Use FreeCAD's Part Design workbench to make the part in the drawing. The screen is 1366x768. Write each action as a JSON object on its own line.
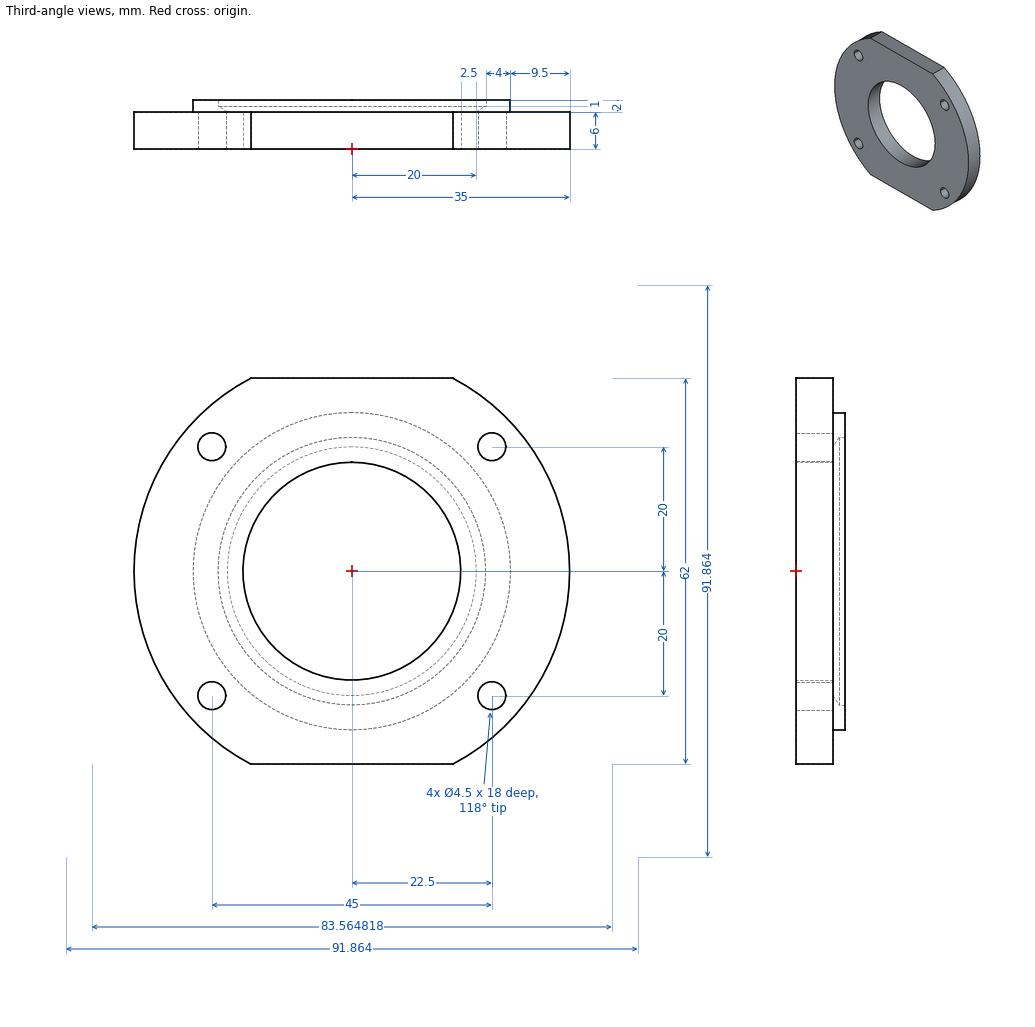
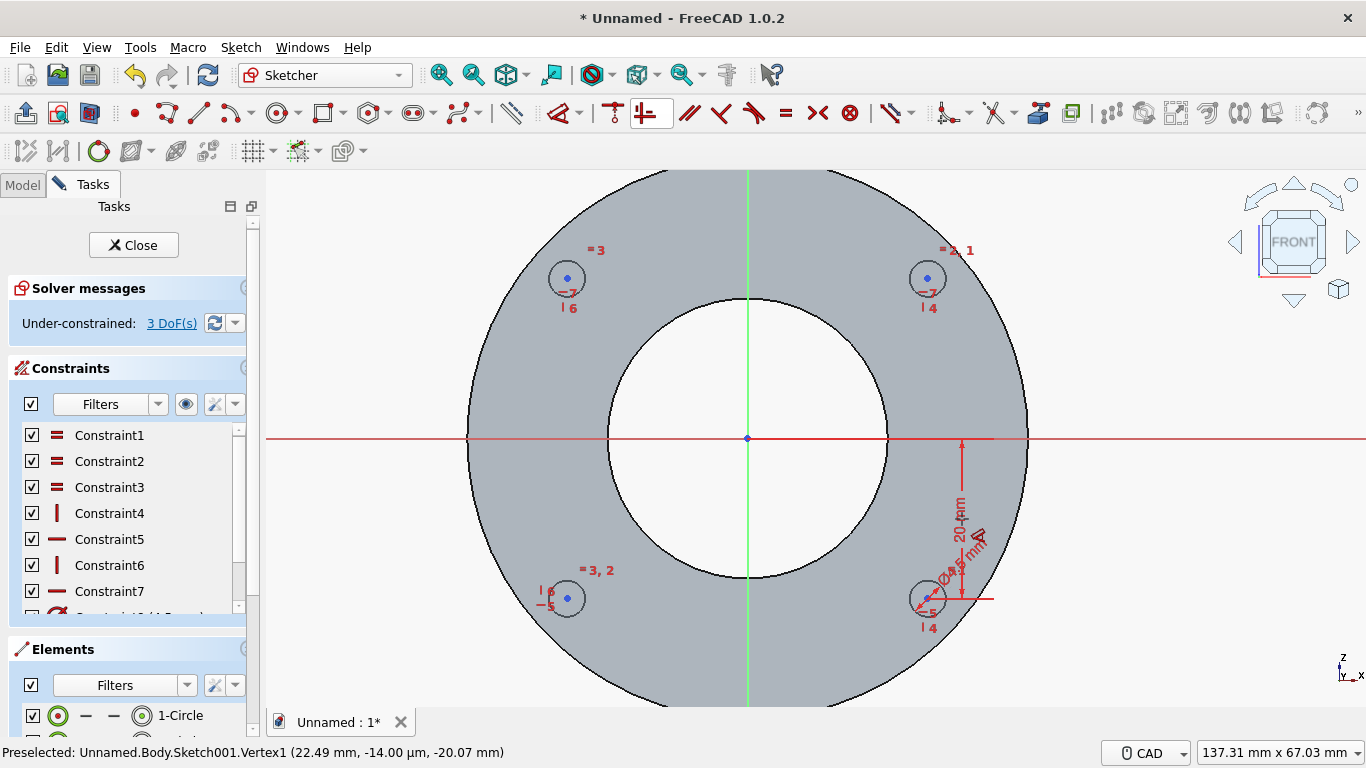
{"action": "left_click", "coordinate": [928, 279]}
{"action": "left_click", "coordinate": [962, 359]}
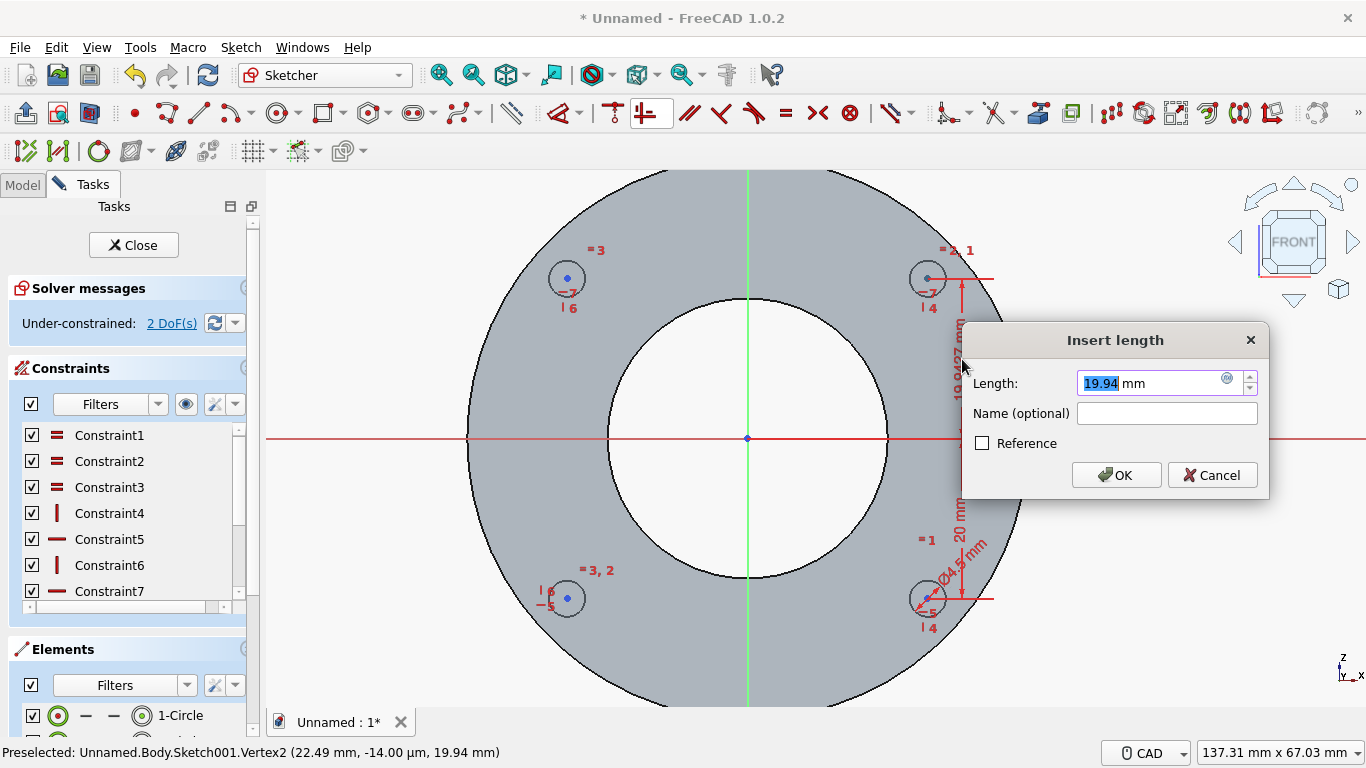
{"action": "type", "text": "20"}
{"action": "key", "text": "Return"}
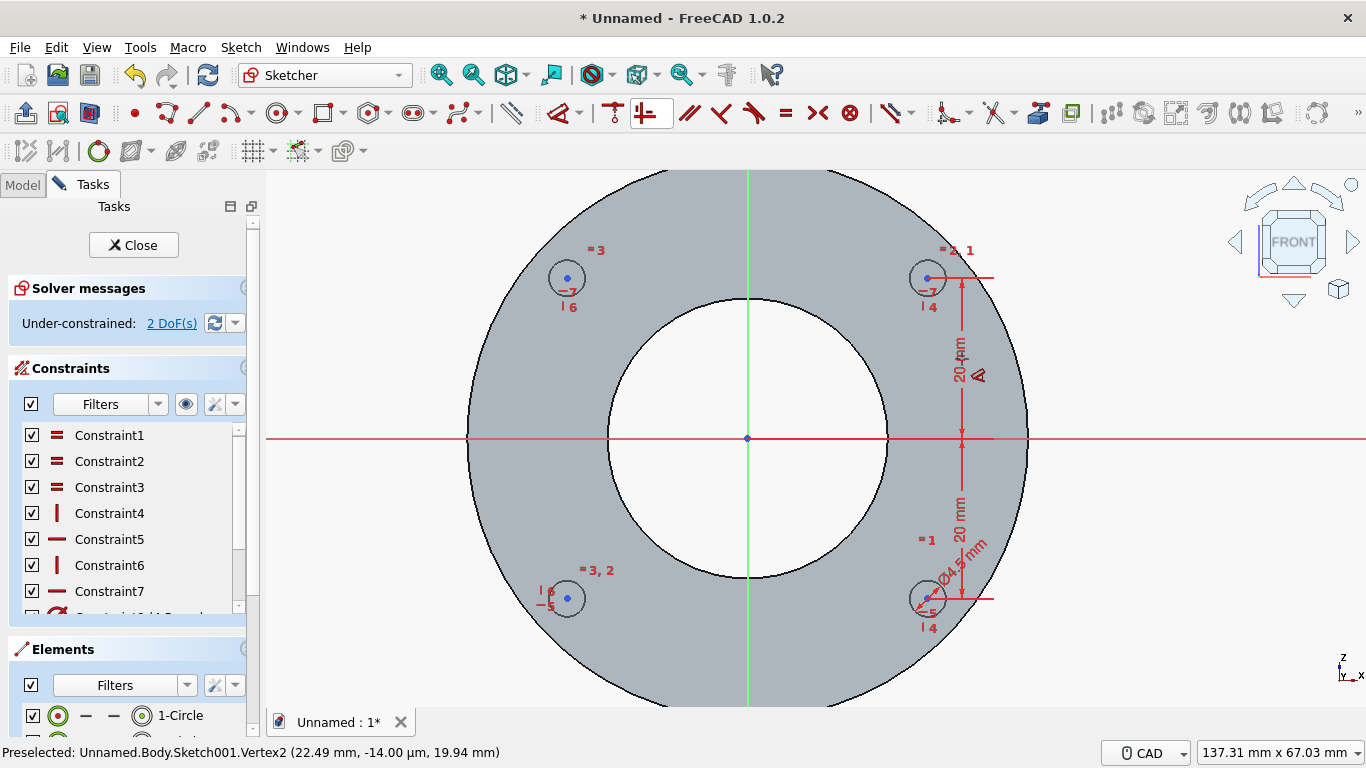
{"action": "left_click", "coordinate": [928, 599]}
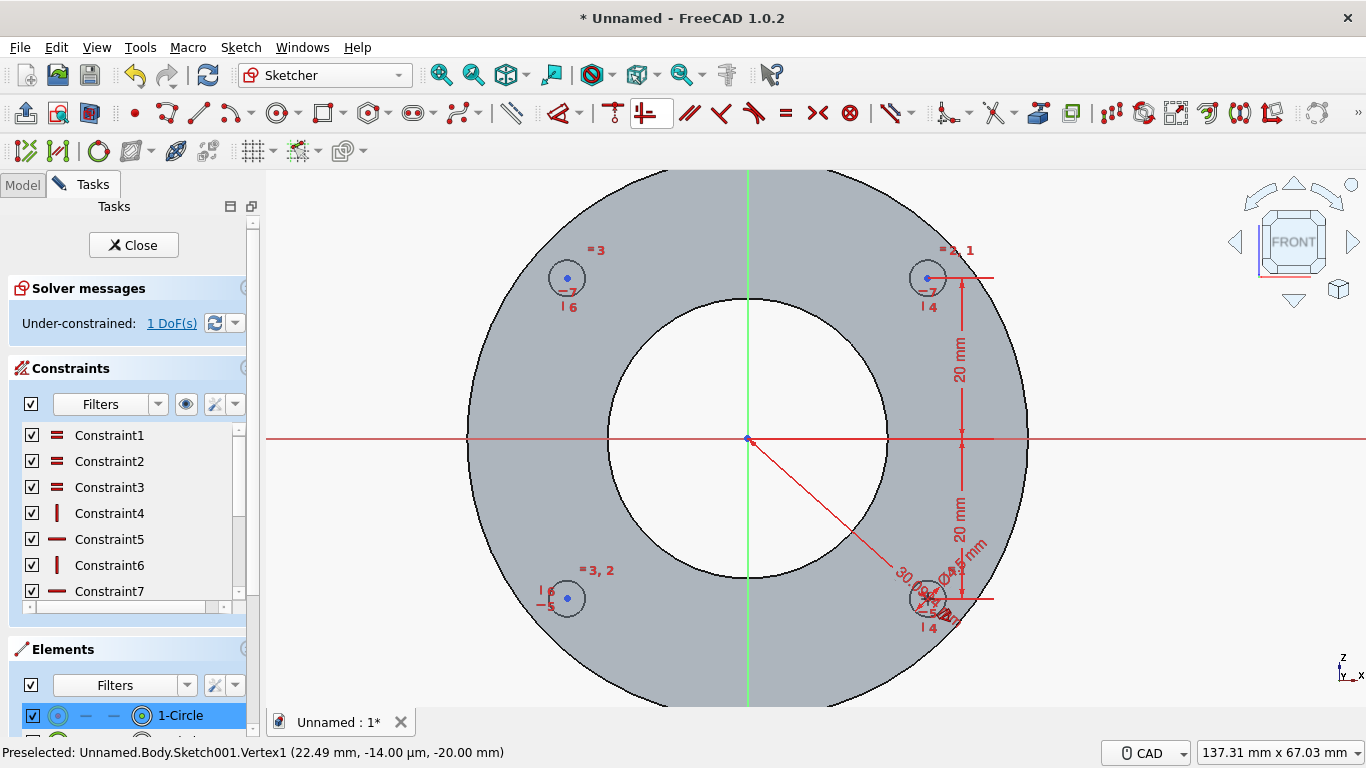
{"action": "left_click", "coordinate": [567, 599]}
{"action": "left_click", "coordinate": [664, 633]}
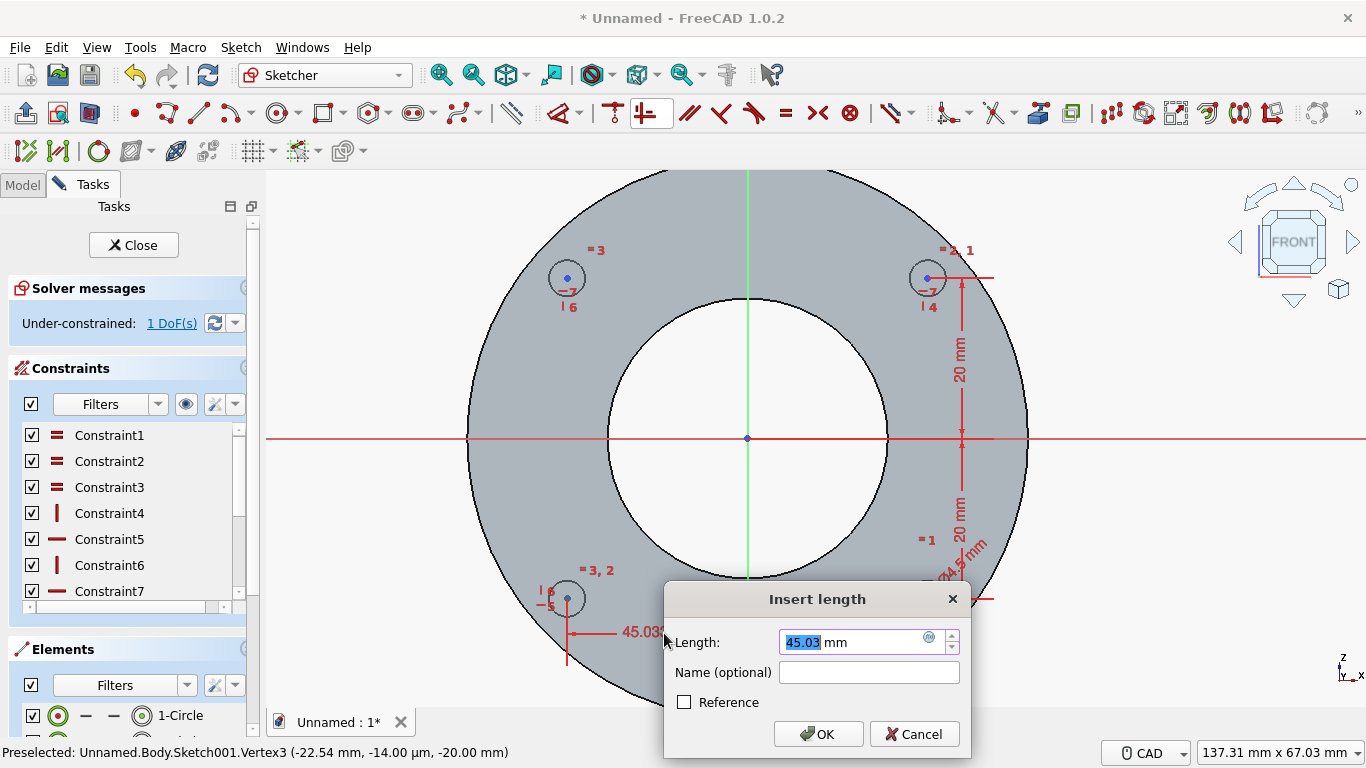
{"action": "type", "text": "45"}
{"action": "key", "text": "Return"}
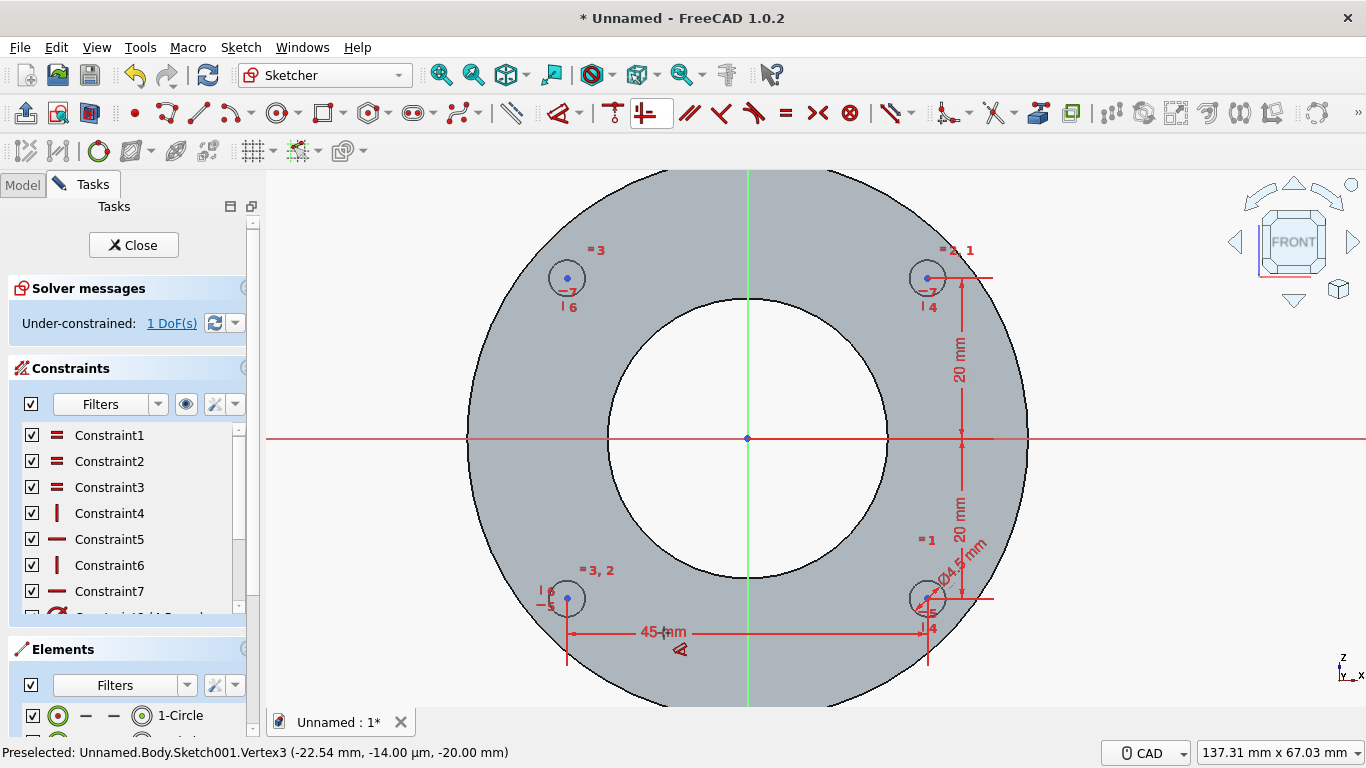
{"action": "left_click", "coordinate": [928, 599]}
{"action": "left_click", "coordinate": [838, 633]}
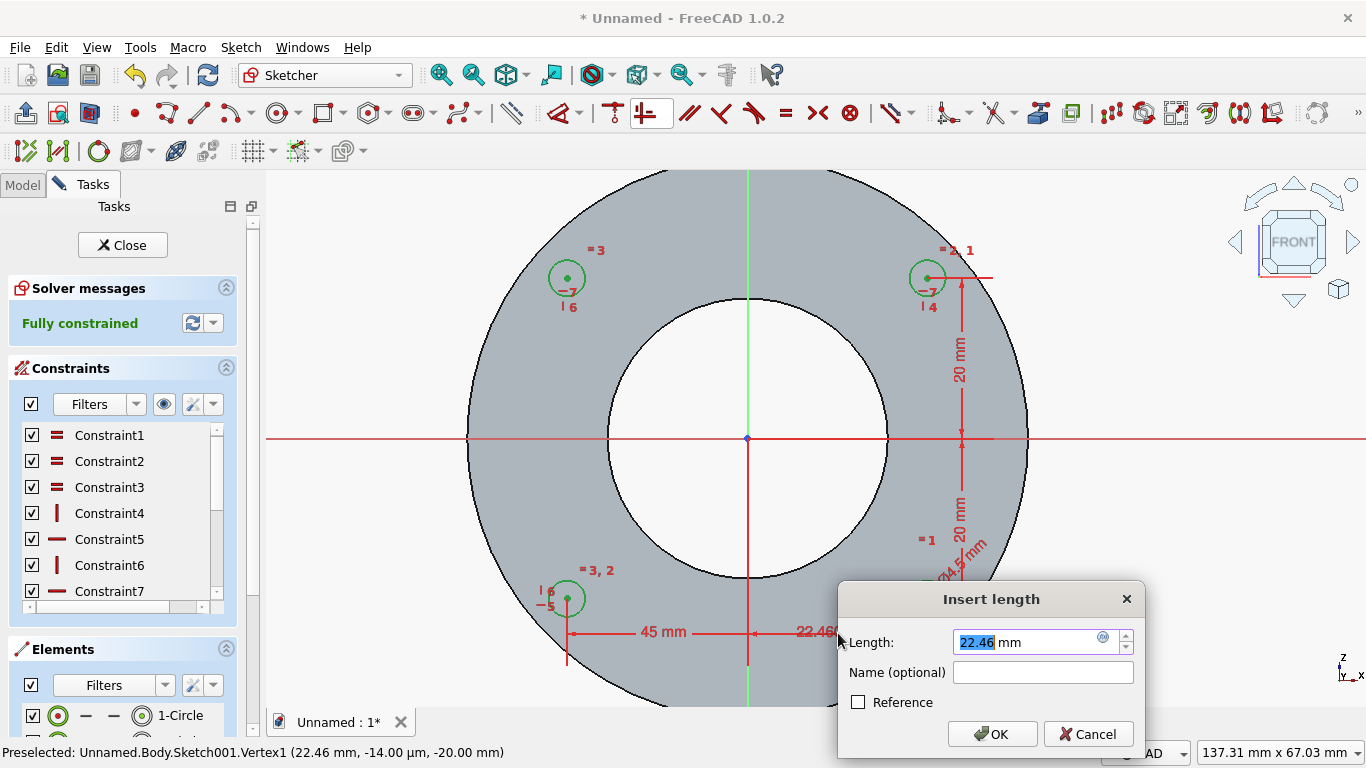
{"action": "type", "text": "22.5"}
{"action": "key", "text": "Return"}
{"action": "key", "text": "Escape"}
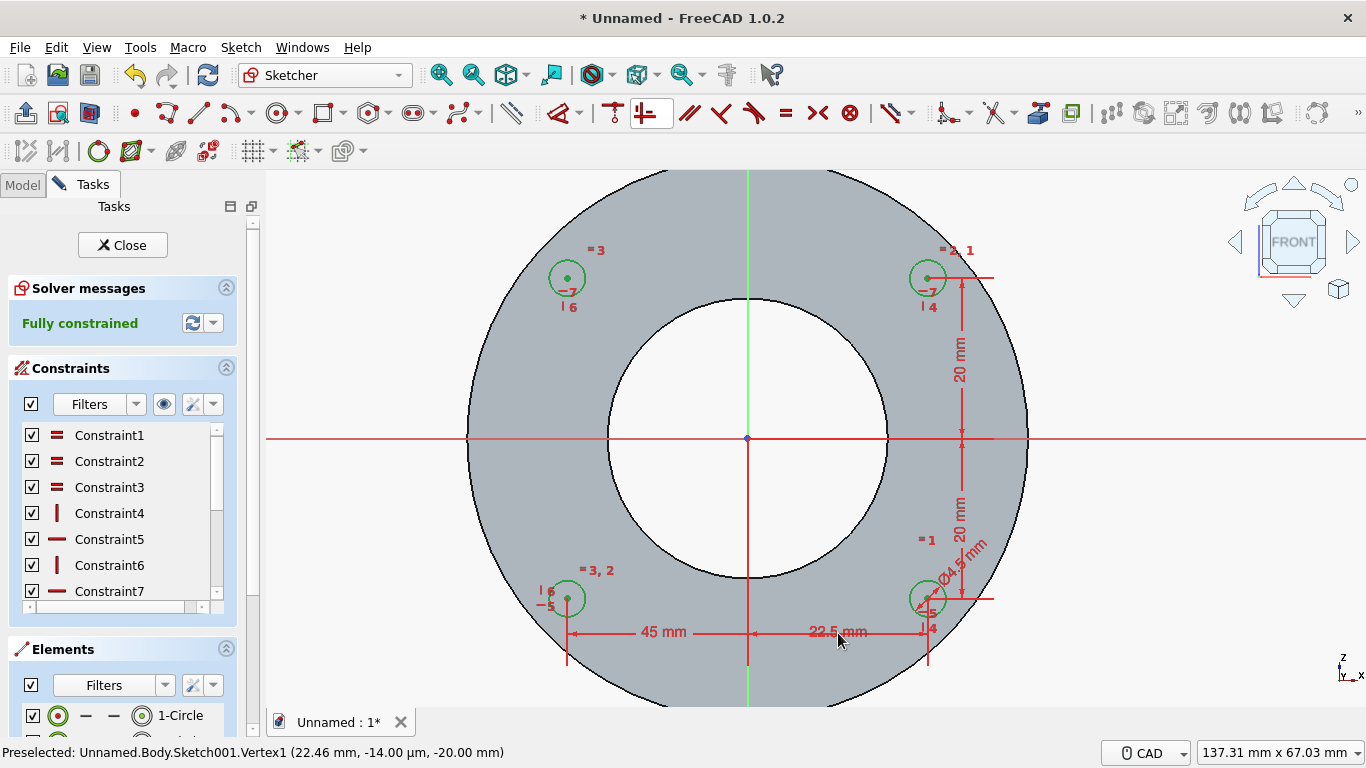
{"action": "left_click", "coordinate": [123, 245]}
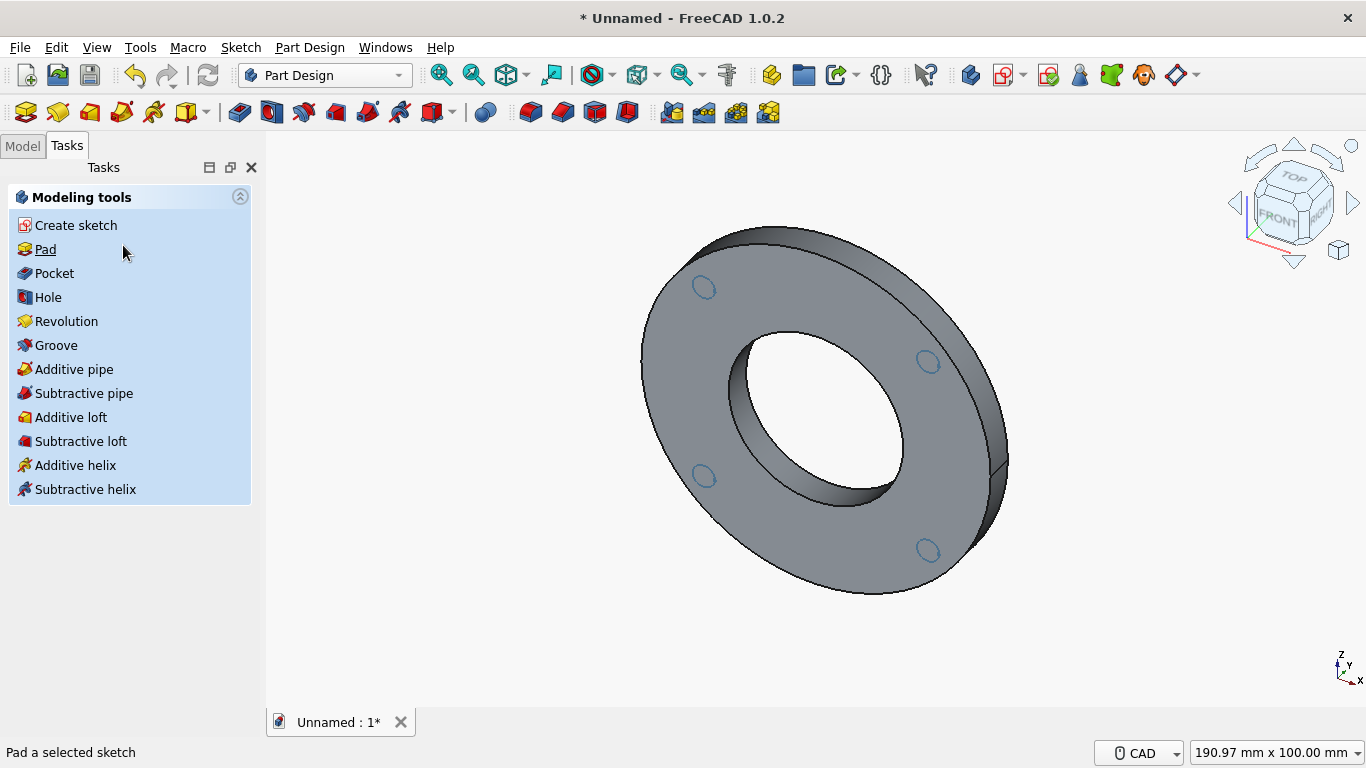
{"action": "left_click", "coordinate": [272, 112]}